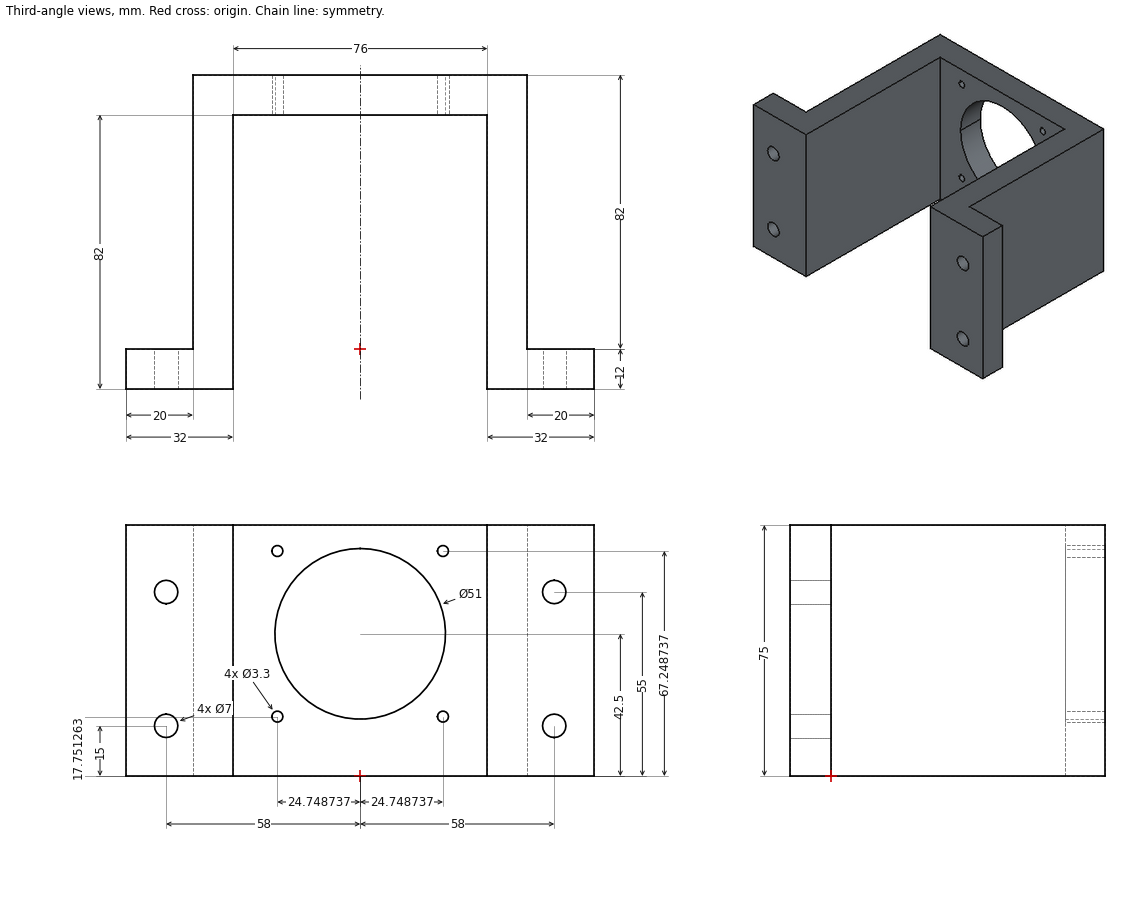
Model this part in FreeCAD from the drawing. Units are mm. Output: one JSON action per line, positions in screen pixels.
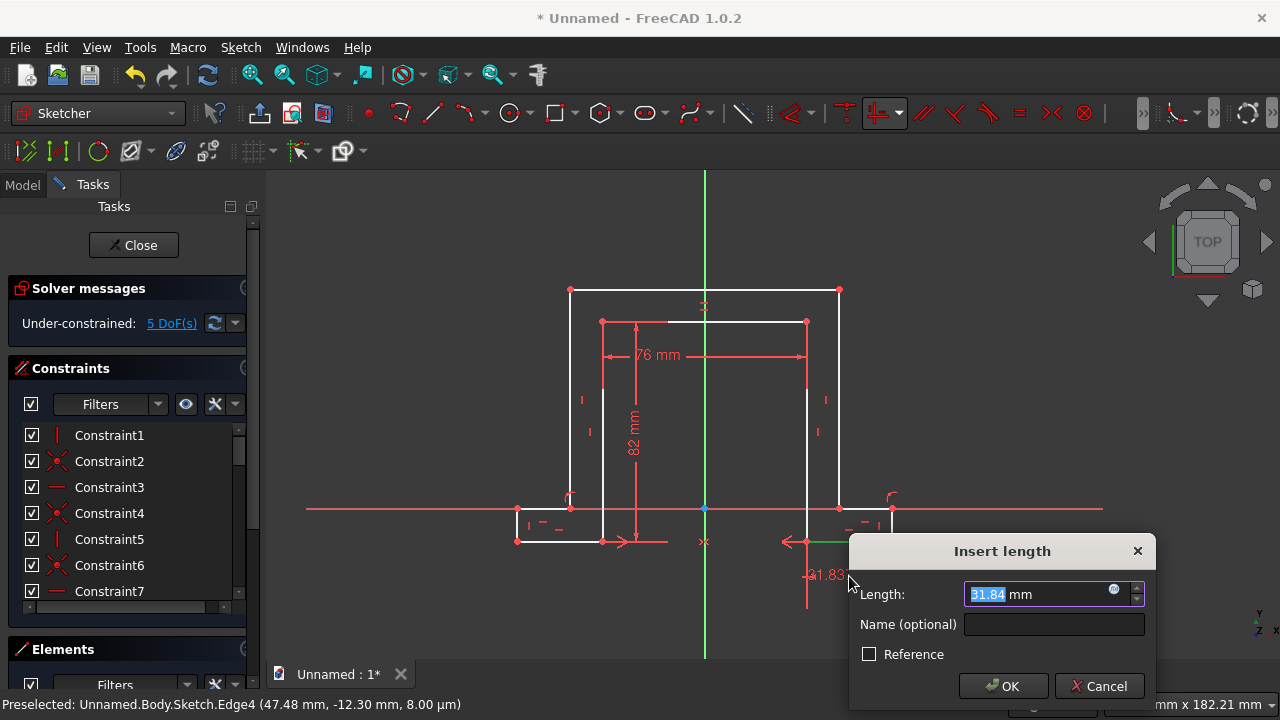
{"action": "type", "text": "32"}
{"action": "key", "text": "Return"}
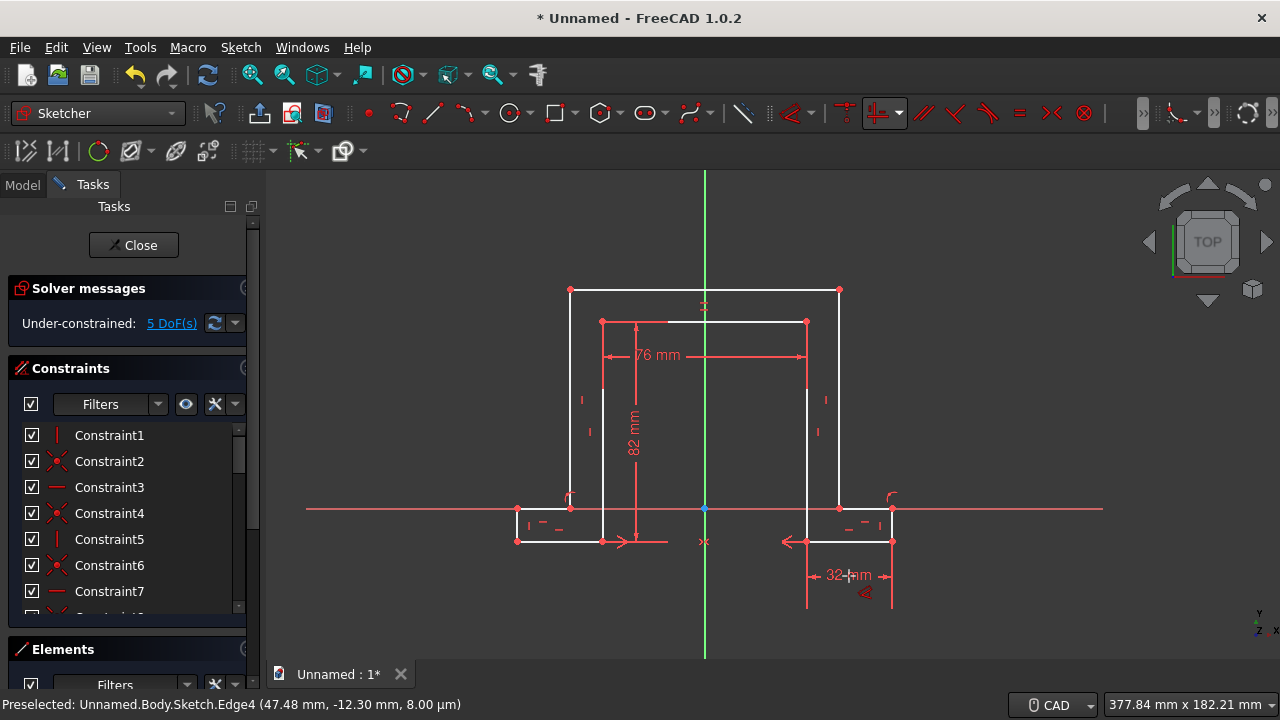
{"action": "scroll", "coordinate": [892, 532], "scroll_direction": "up", "scroll_amount": 2}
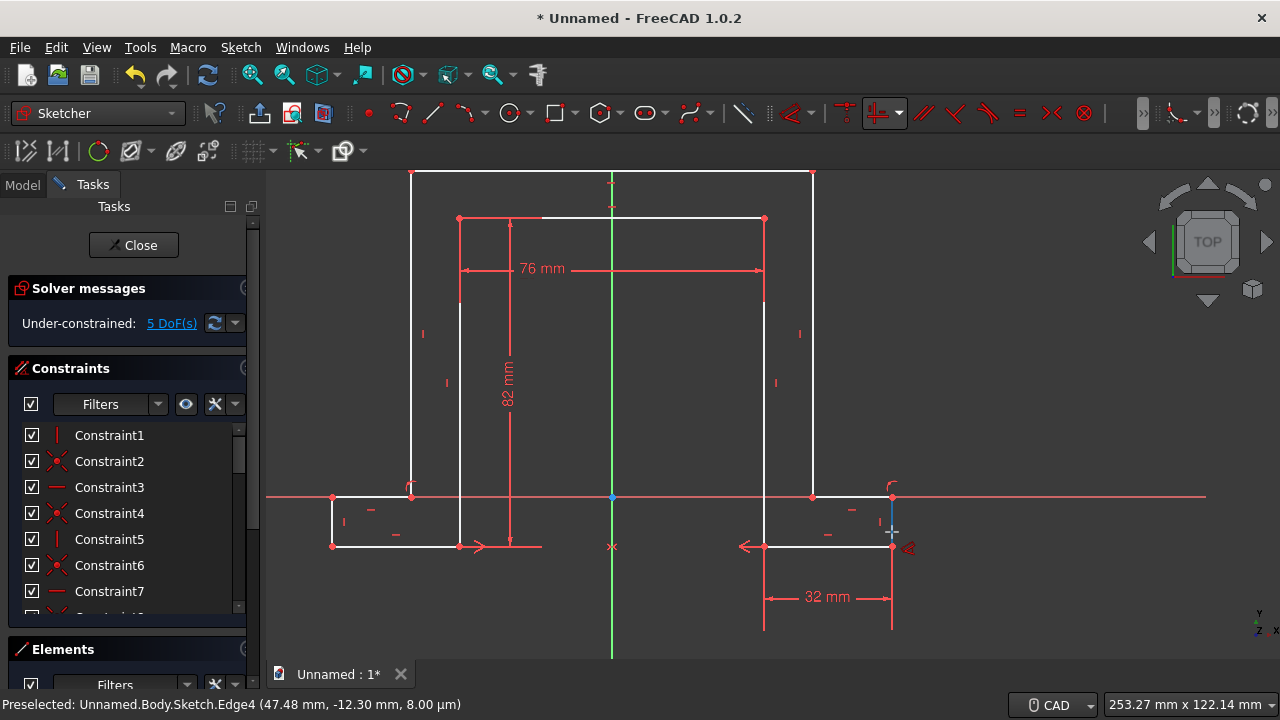
{"action": "left_click", "coordinate": [892, 532]}
{"action": "left_click", "coordinate": [926, 522]}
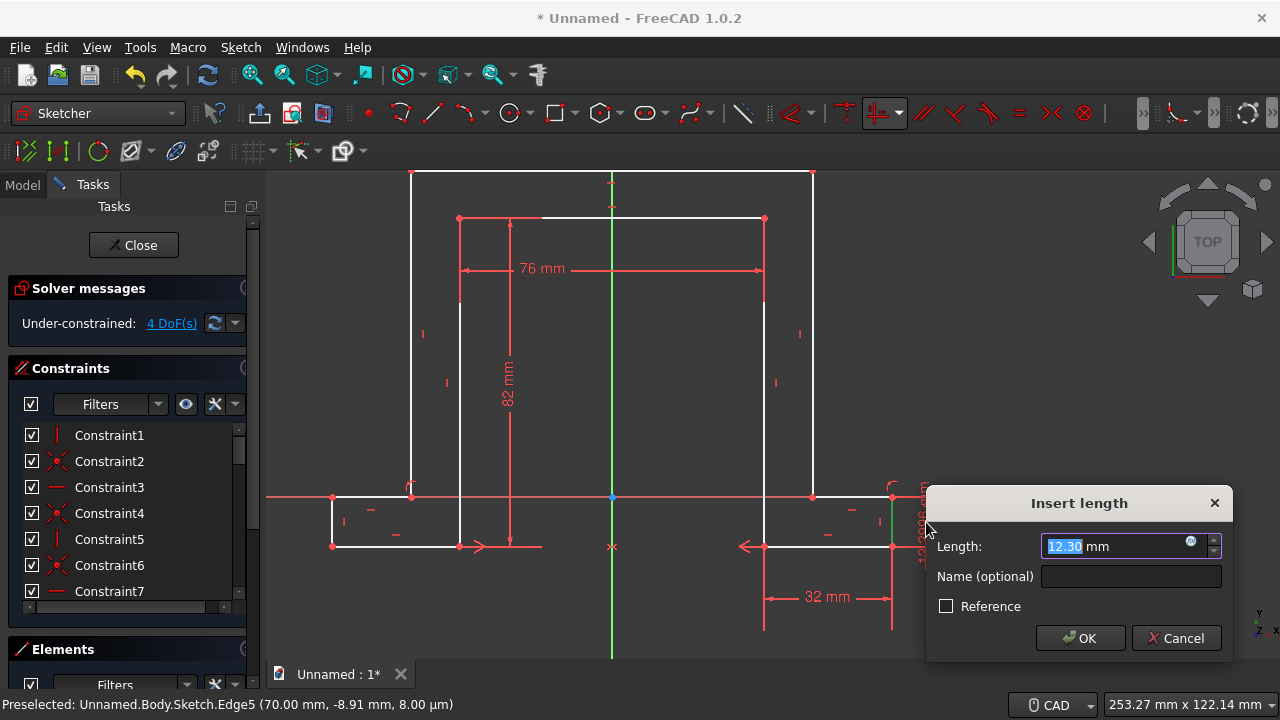
{"action": "type", "text": "12"}
{"action": "key", "text": "Return"}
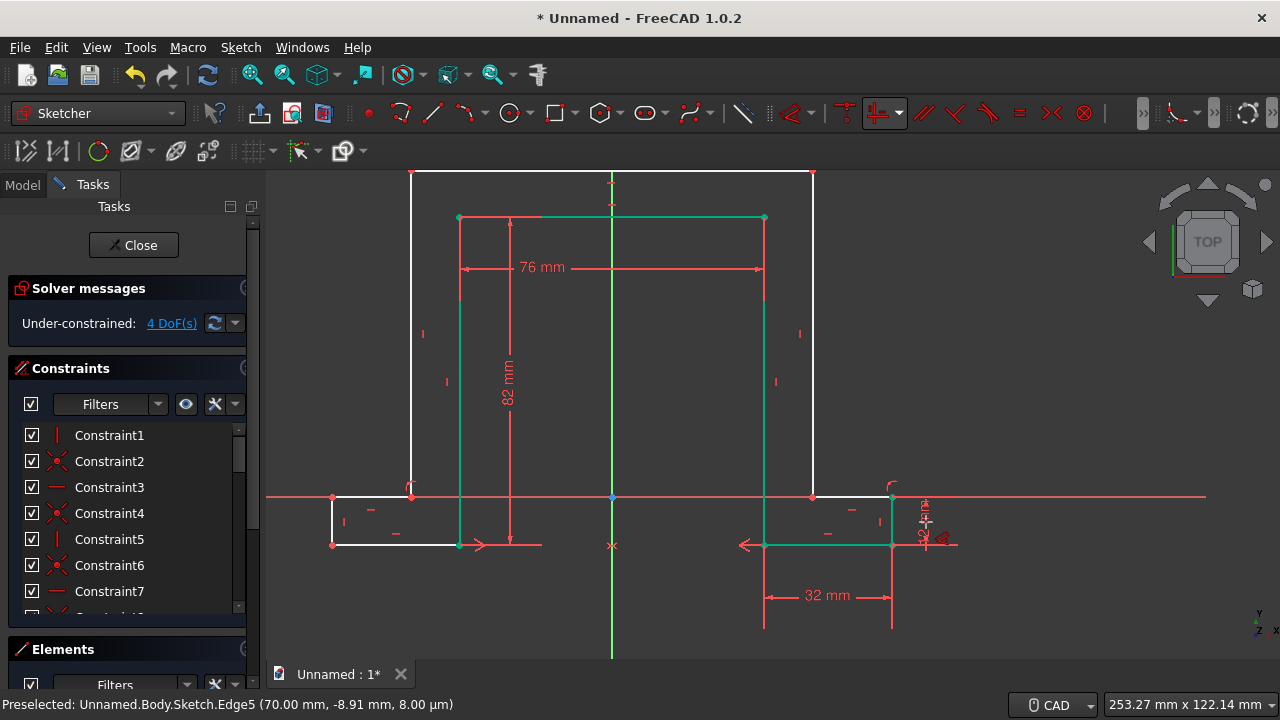
{"action": "left_click", "coordinate": [868, 497]}
{"action": "left_click", "coordinate": [852, 531]}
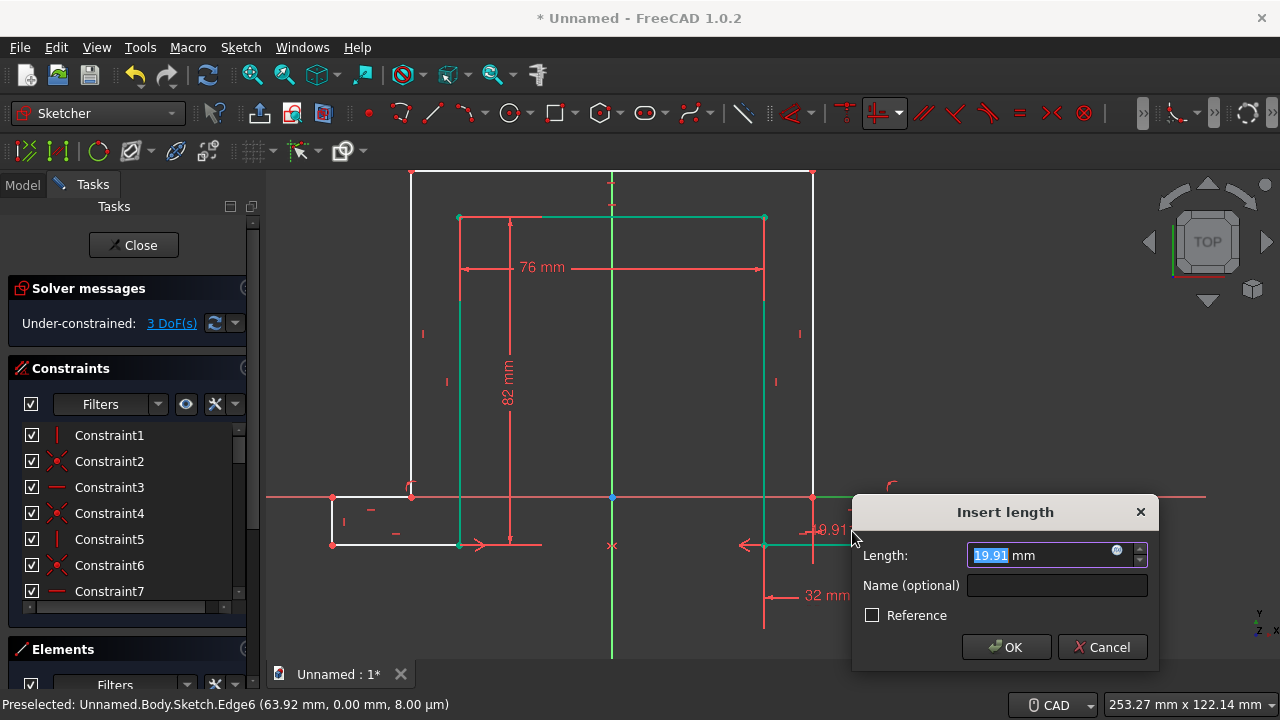
{"action": "type", "text": "20"}
{"action": "key", "text": "Return"}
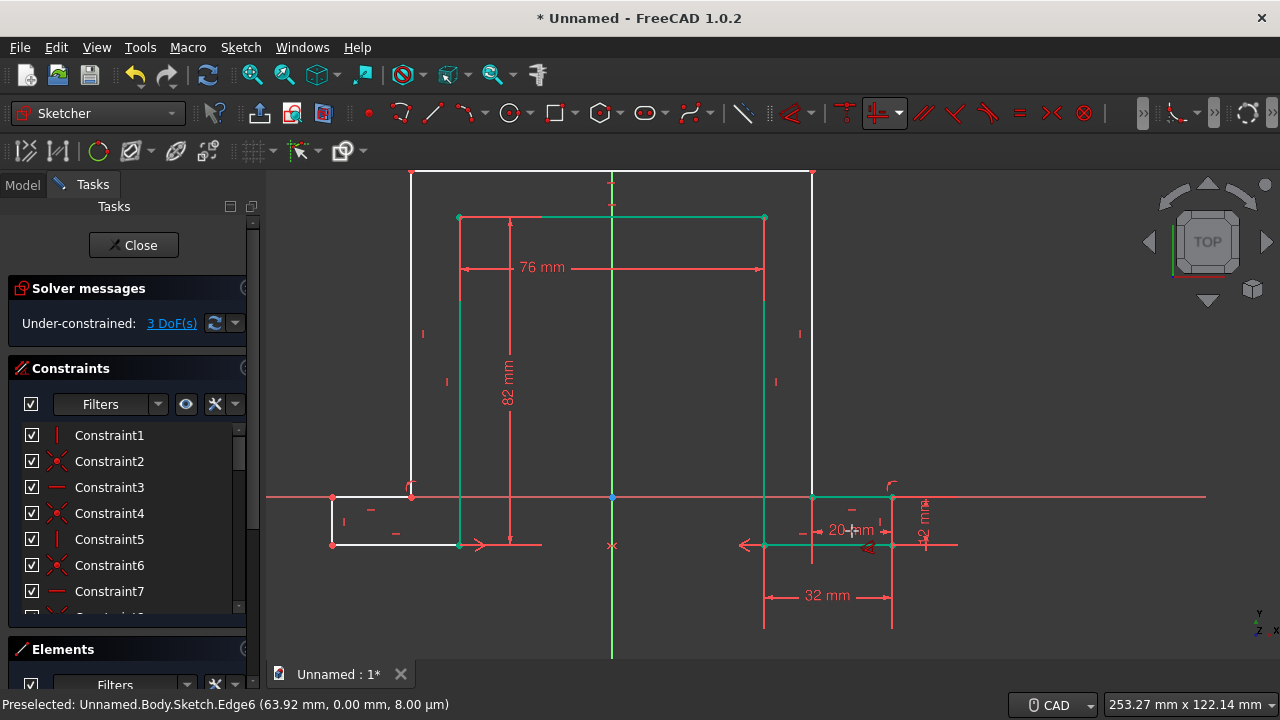
{"action": "left_click", "coordinate": [812, 399]}
{"action": "left_click", "coordinate": [846, 348]}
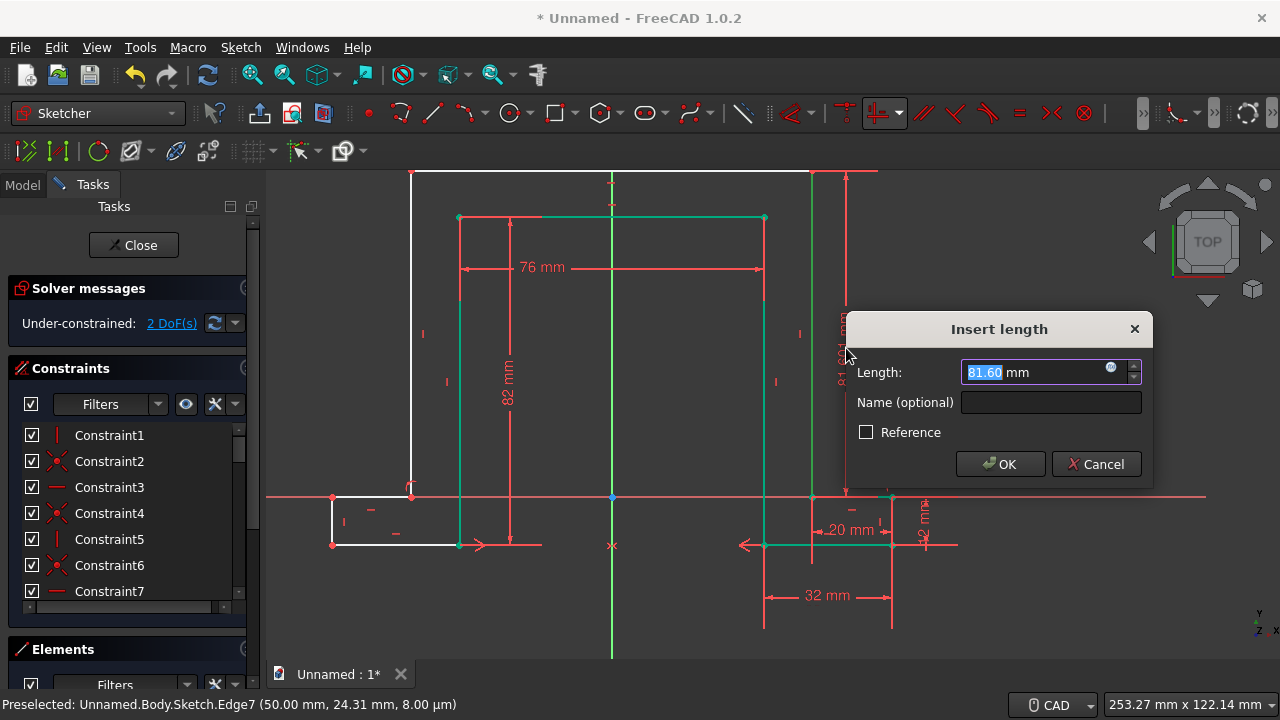
{"action": "type", "text": "82"}
{"action": "key", "text": "Return"}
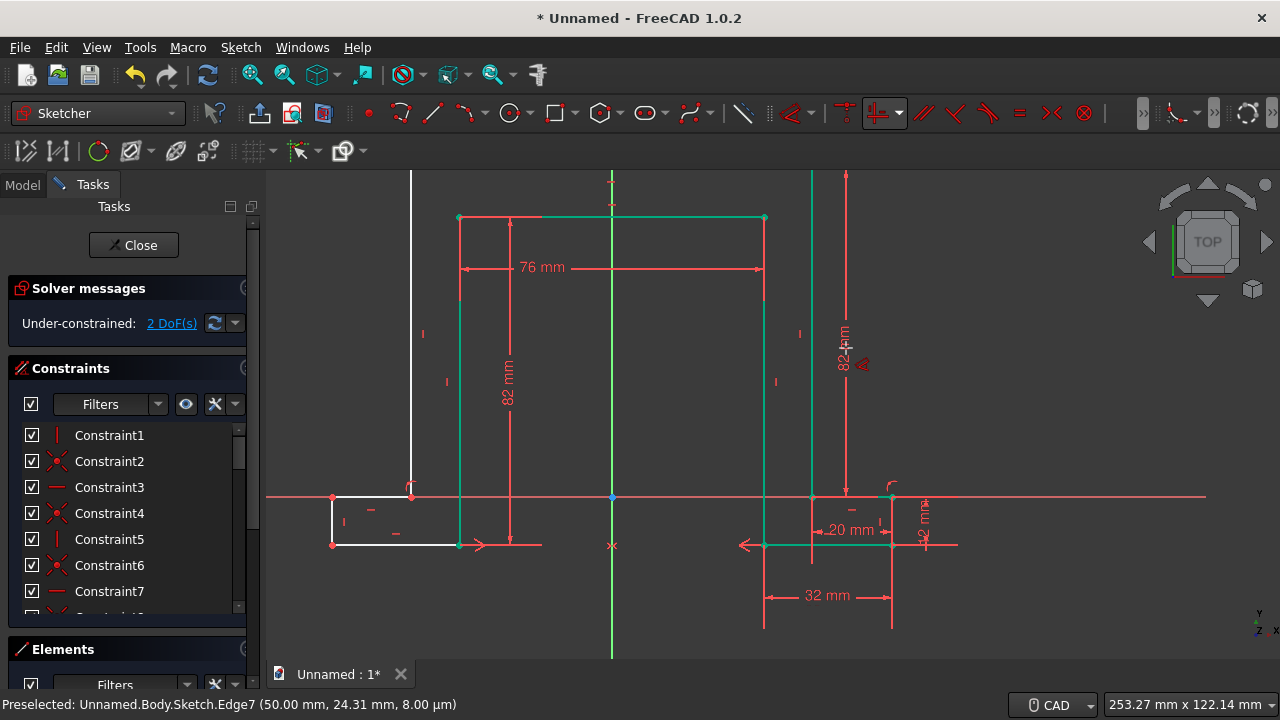
{"action": "left_click", "coordinate": [388, 497]}
{"action": "left_click", "coordinate": [372, 531]}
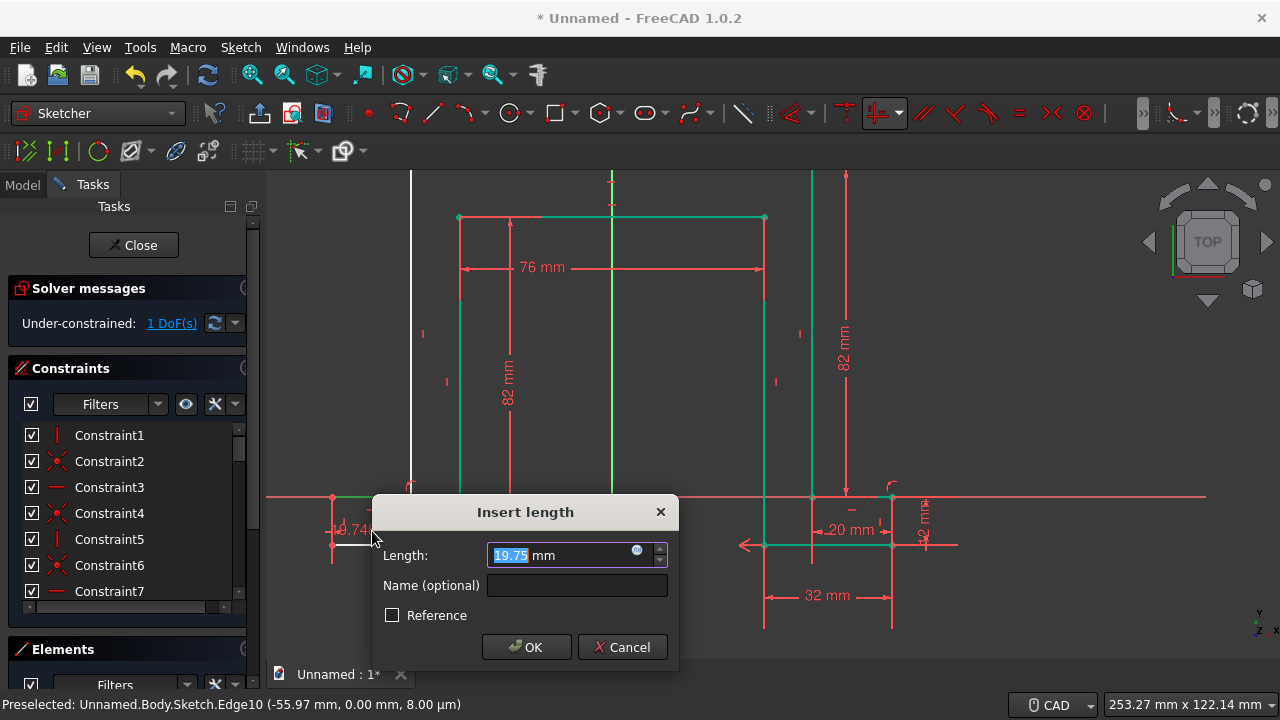
{"action": "type", "text": "20"}
{"action": "key", "text": "Return"}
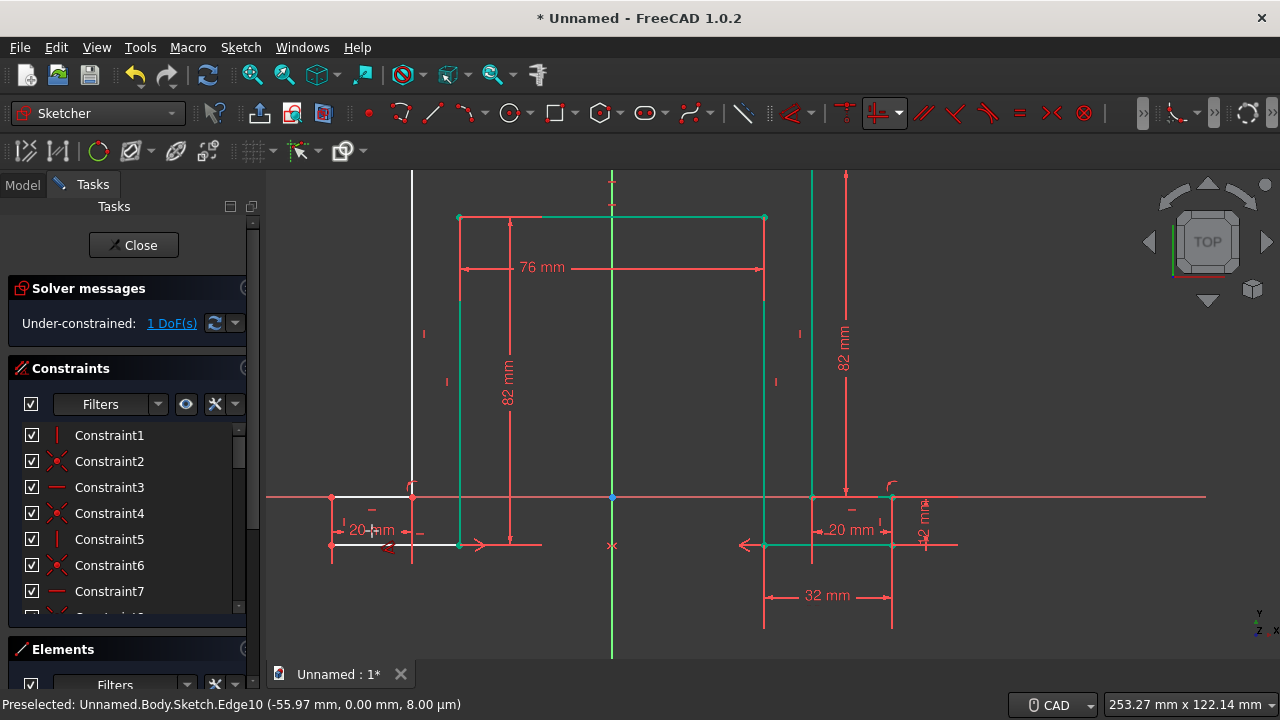
{"action": "left_click", "coordinate": [370, 545]}
{"action": "left_click", "coordinate": [396, 579]}